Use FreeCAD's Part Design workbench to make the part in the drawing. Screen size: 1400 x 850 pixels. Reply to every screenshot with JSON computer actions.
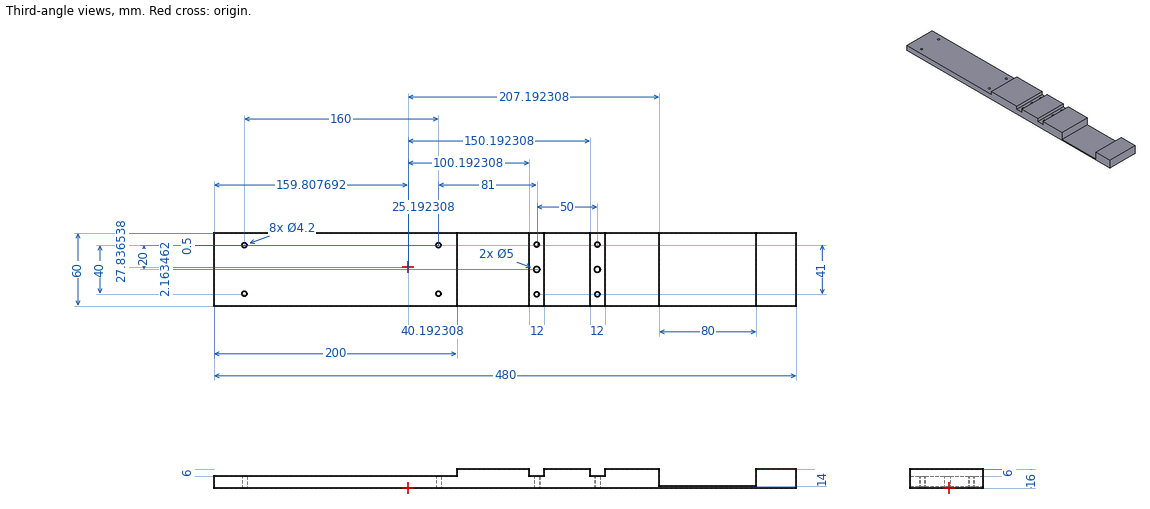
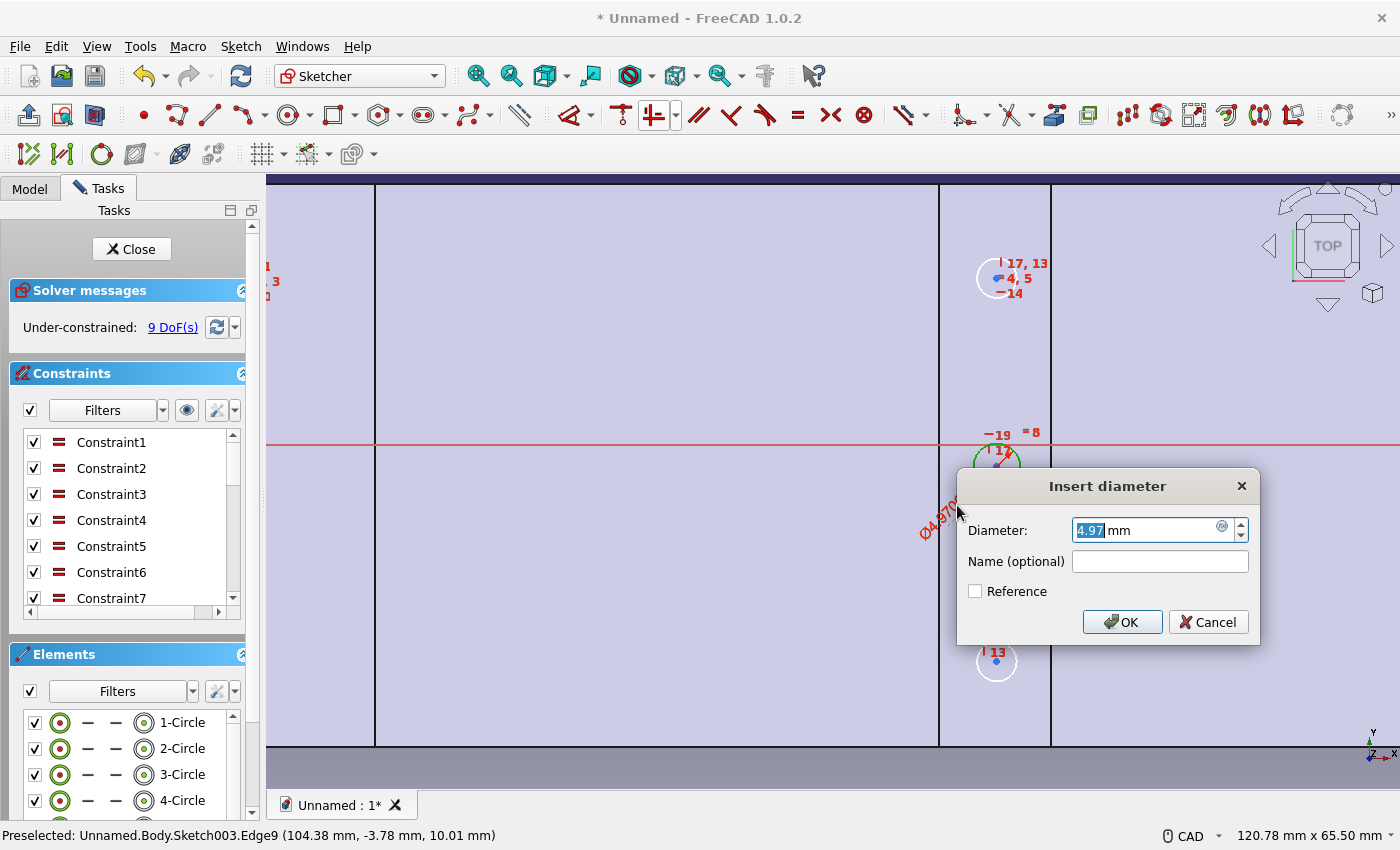
{"action": "type", "text": "5"}
{"action": "key", "text": "Return"}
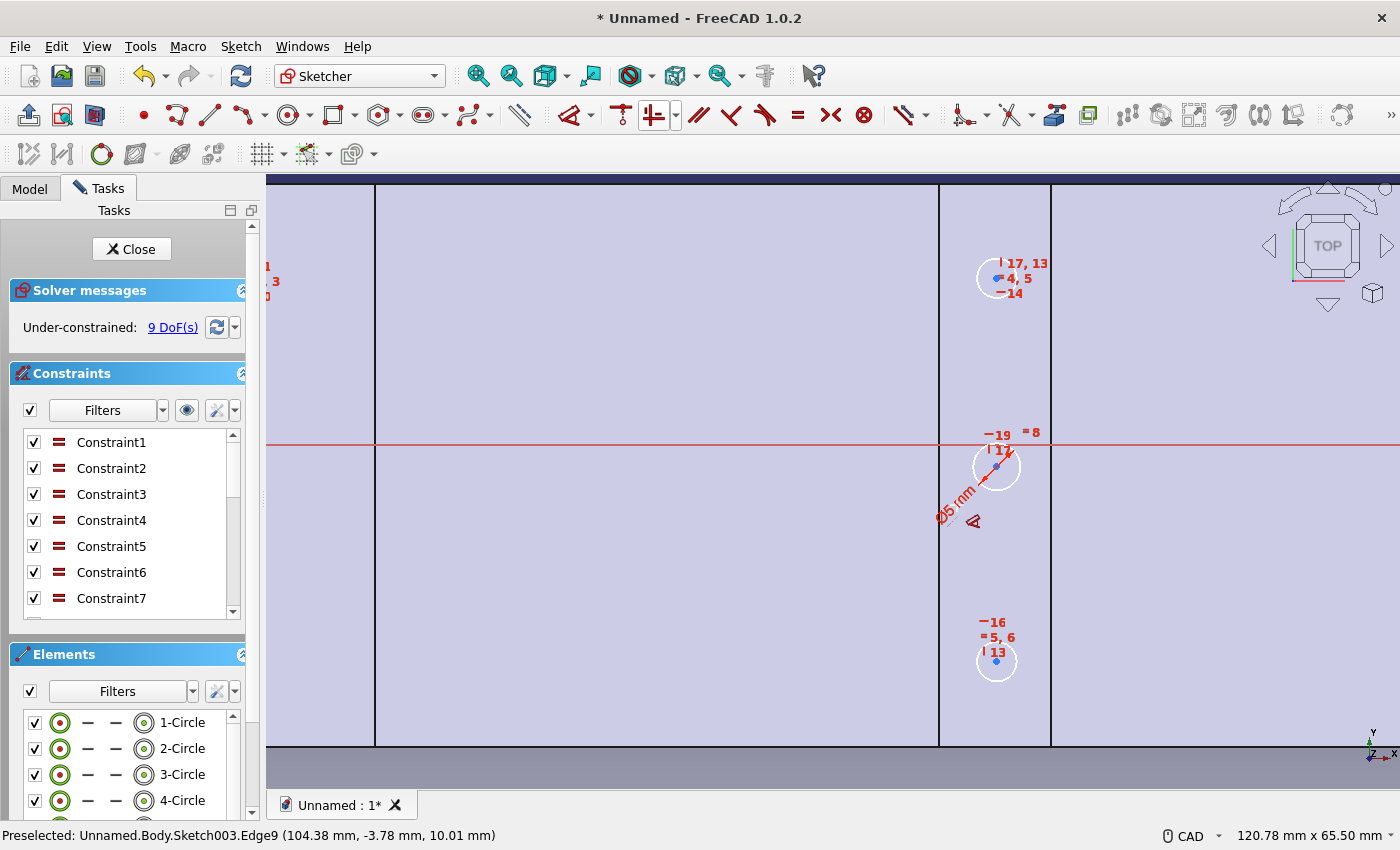
{"action": "scroll", "coordinate": [982, 487], "scroll_direction": "down", "scroll_amount": 7}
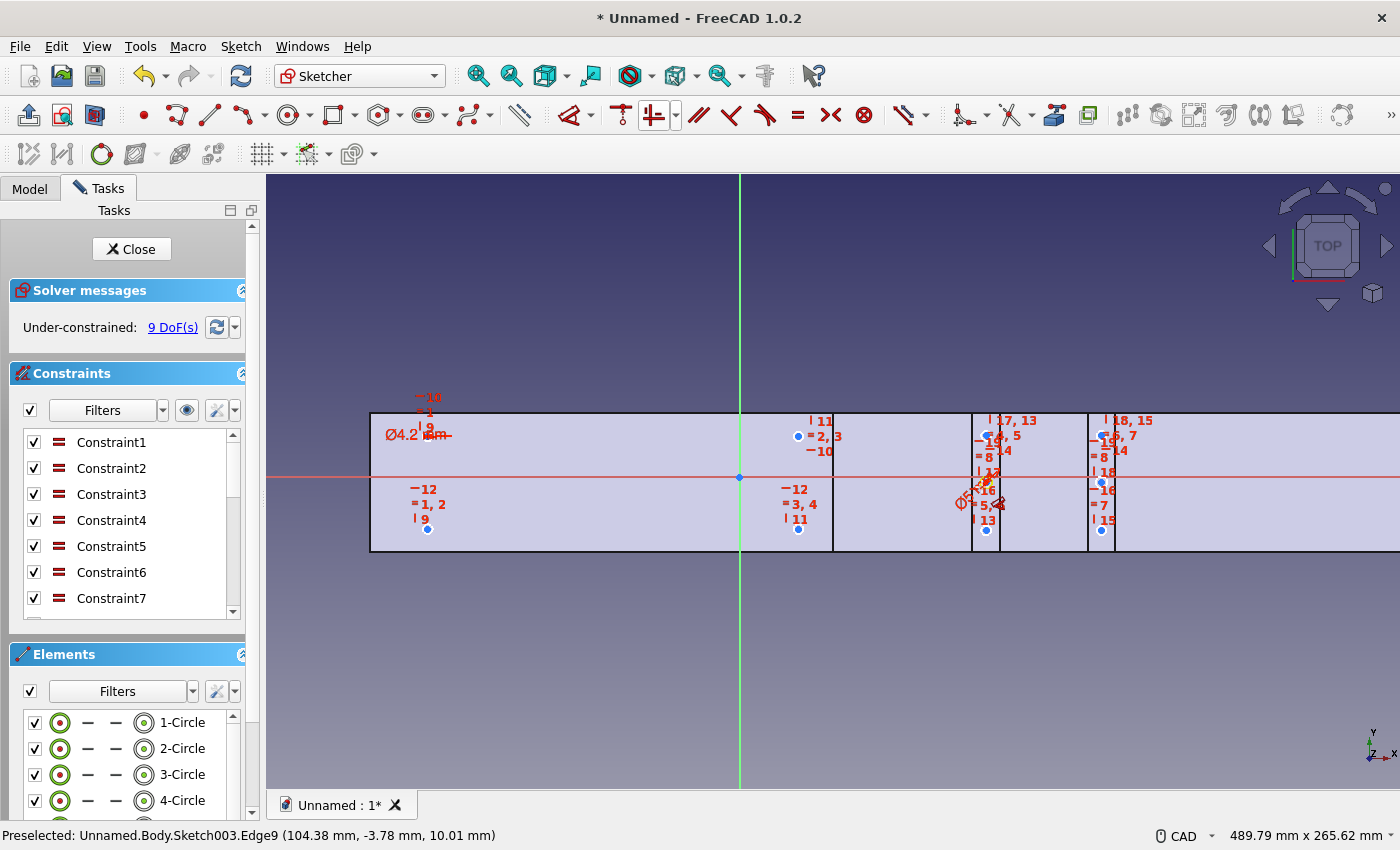
{"action": "left_click", "coordinate": [428, 437]}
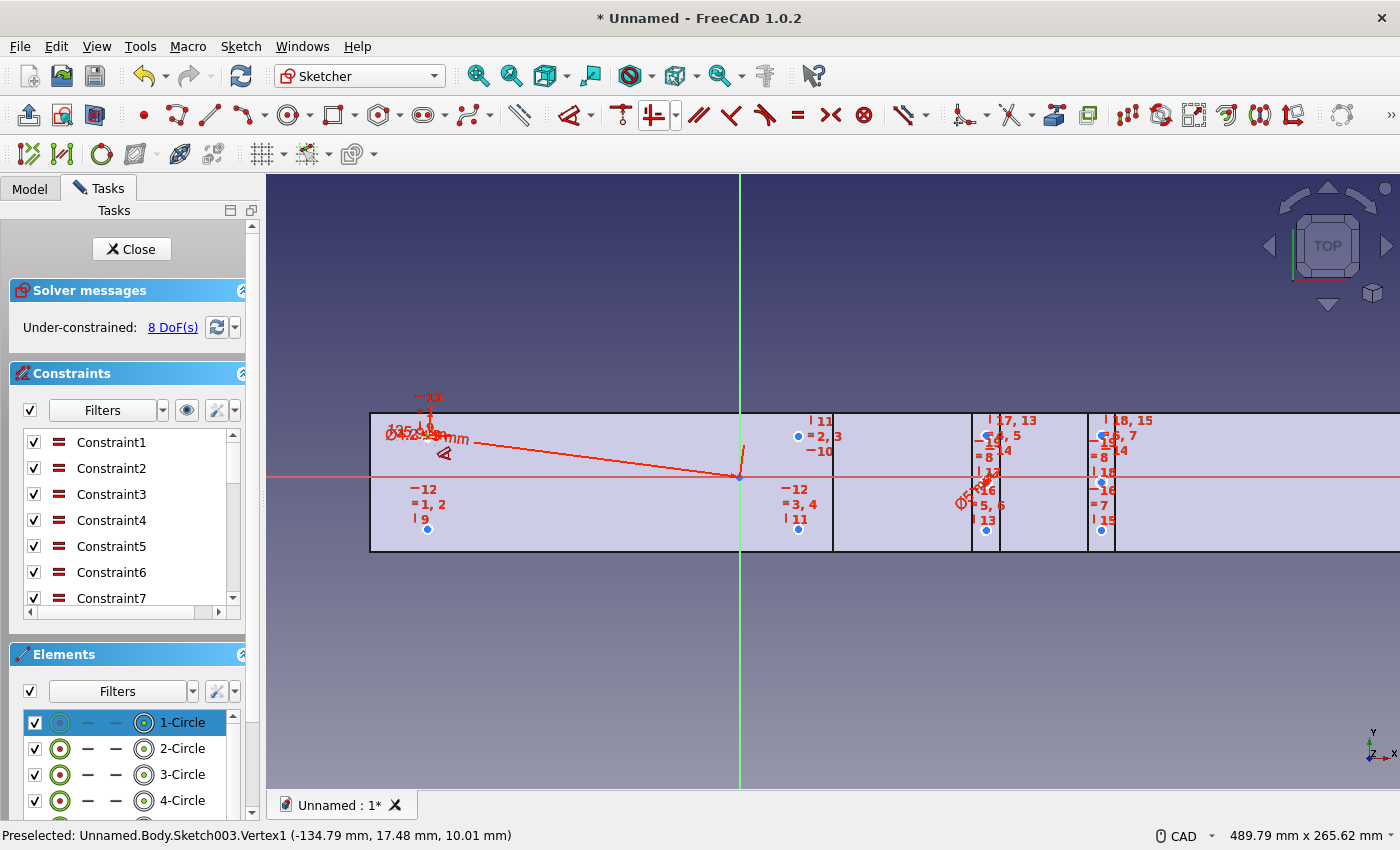
{"action": "left_click", "coordinate": [428, 529]}
{"action": "left_click", "coordinate": [394, 462]}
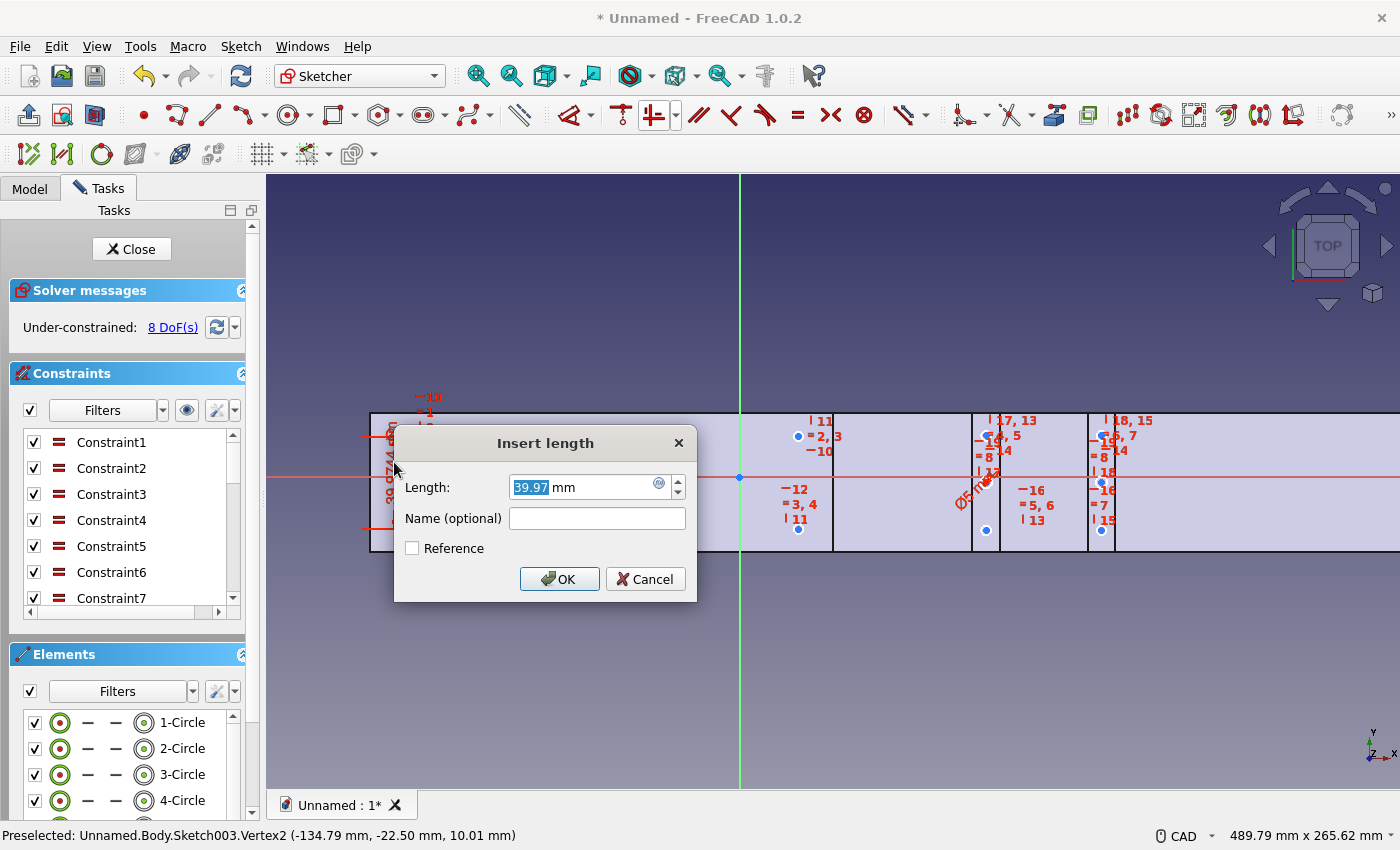
{"action": "type", "text": "40"}
{"action": "key", "text": "Return"}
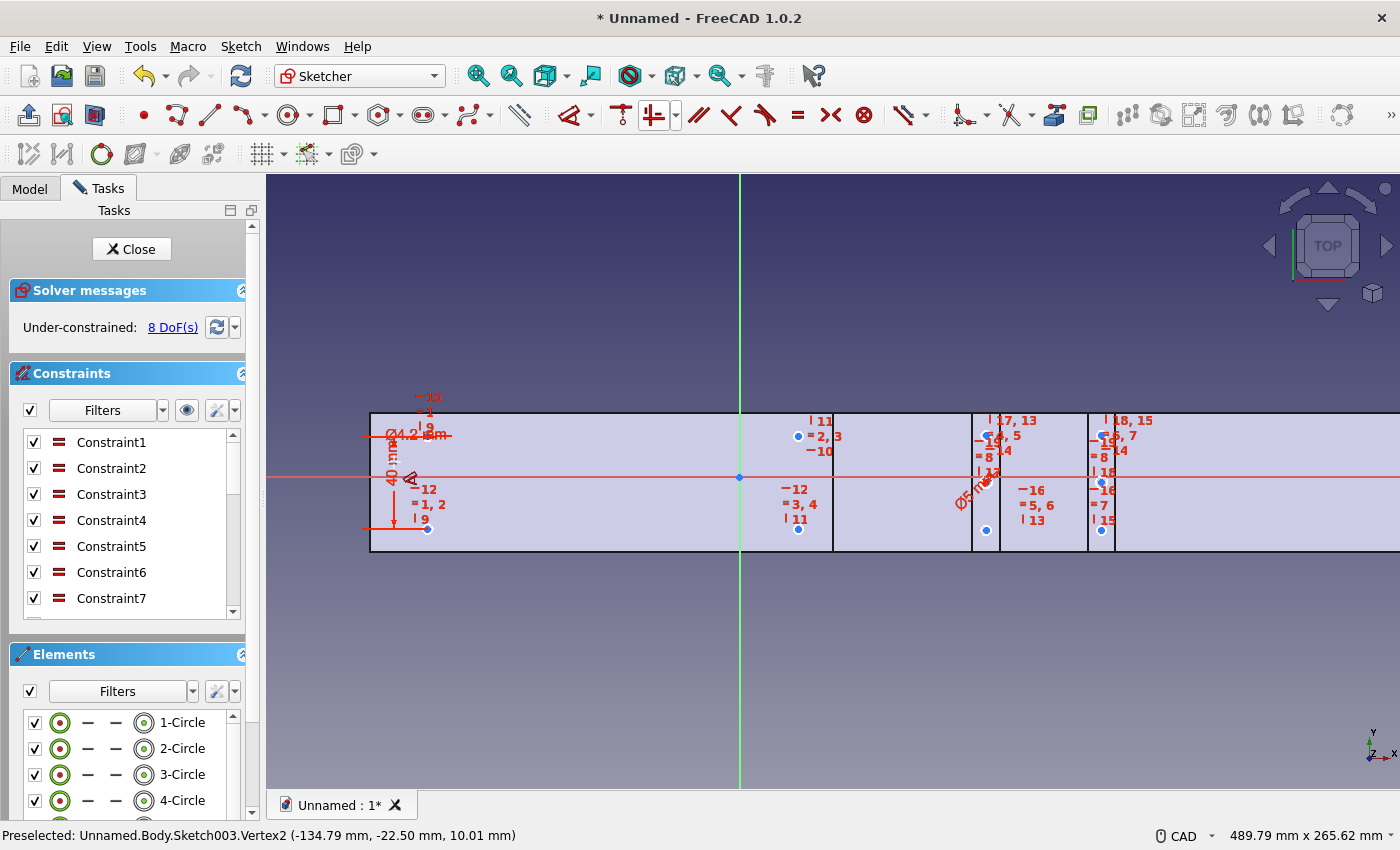
{"action": "left_click", "coordinate": [799, 437]}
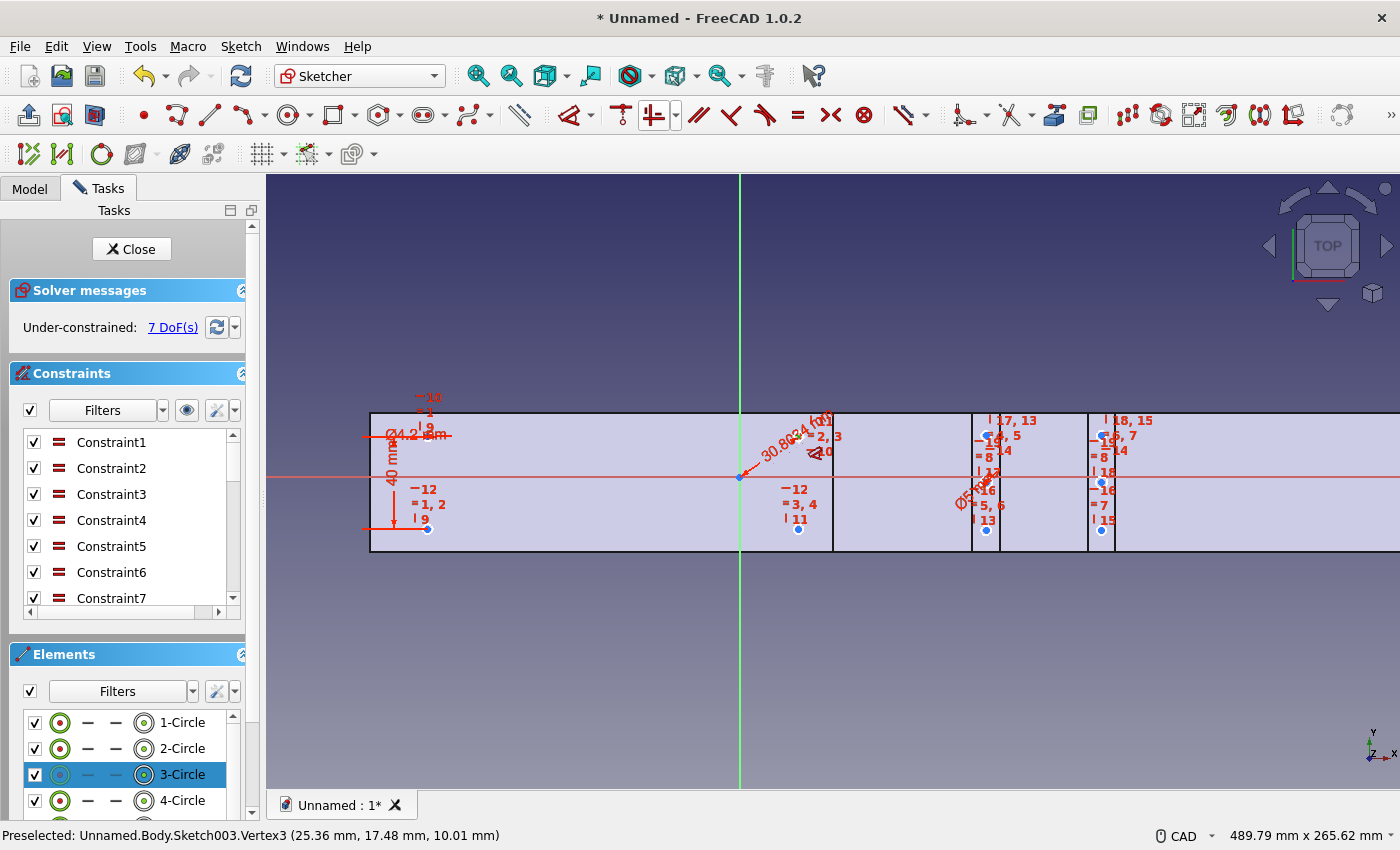
{"action": "left_click", "coordinate": [986, 436]}
{"action": "left_click", "coordinate": [892, 402]}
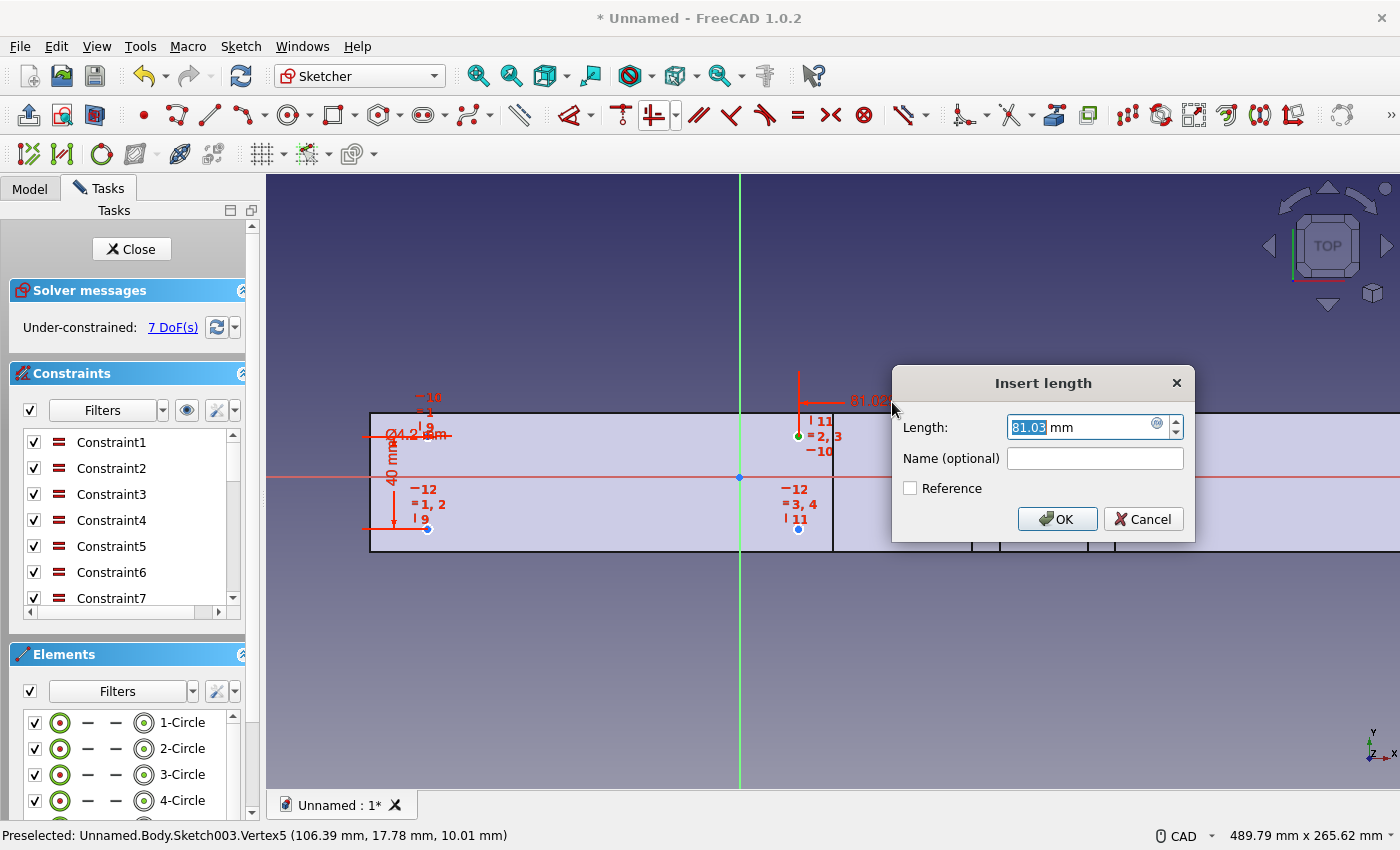
{"action": "type", "text": "81"}
{"action": "key", "text": "Return"}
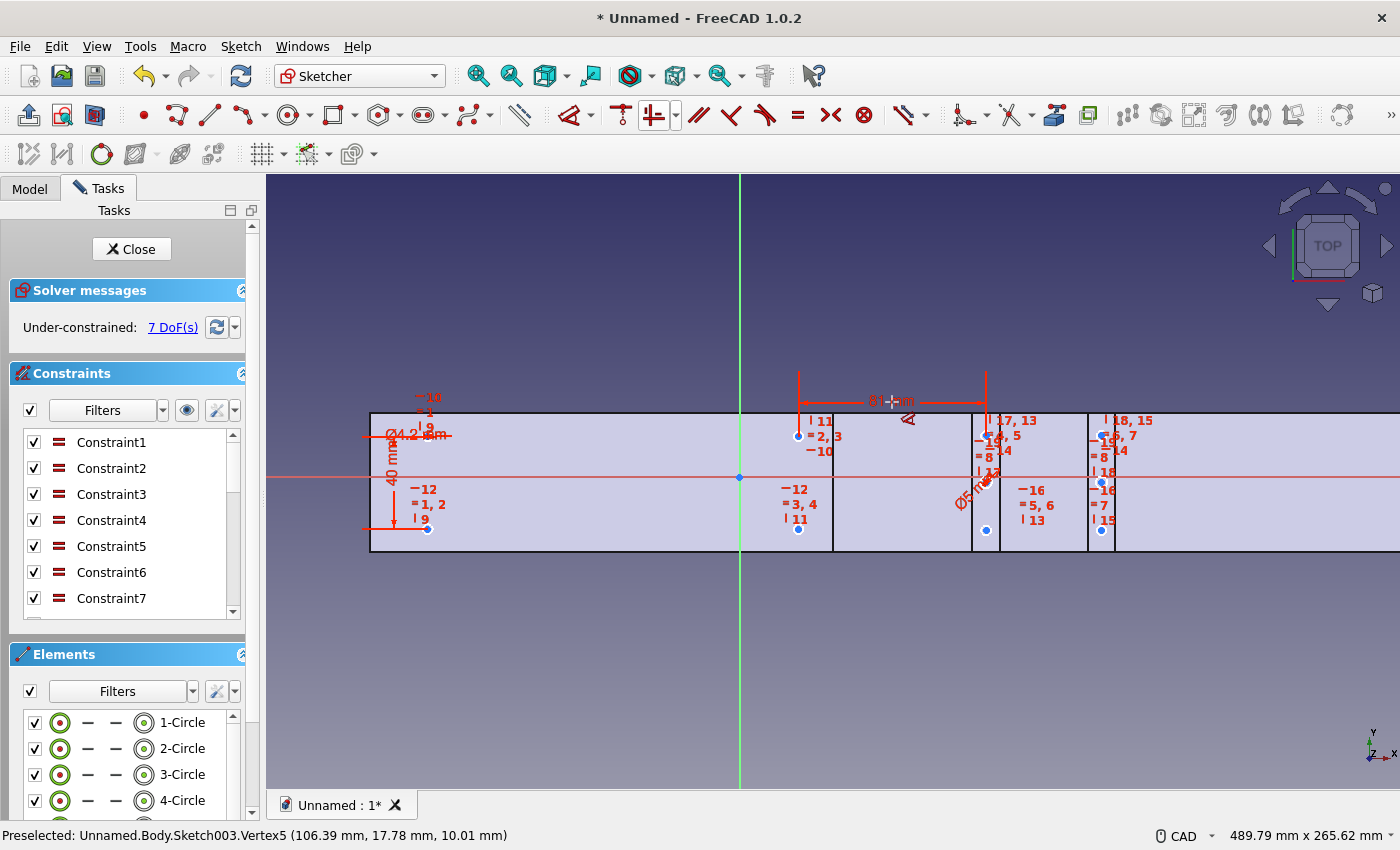
{"action": "left_click", "coordinate": [986, 436]}